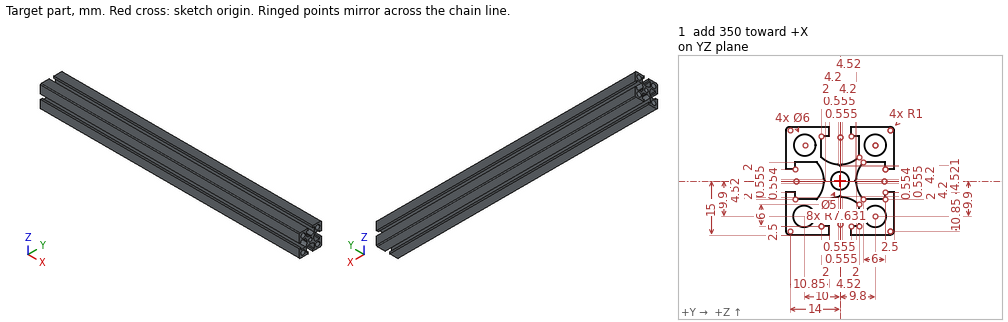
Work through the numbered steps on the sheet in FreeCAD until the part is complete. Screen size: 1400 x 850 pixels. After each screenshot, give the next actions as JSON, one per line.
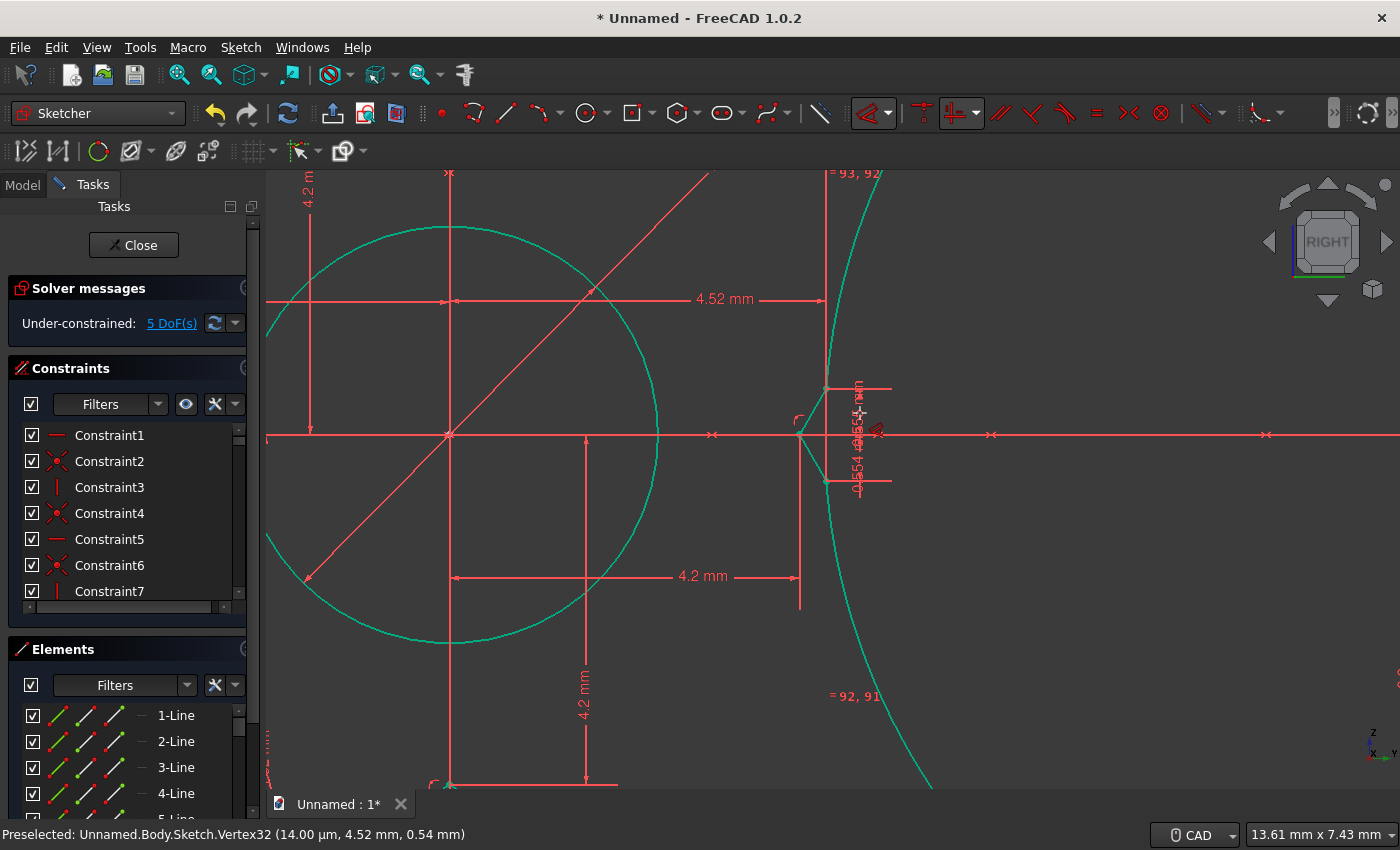
{"action": "scroll", "coordinate": [827, 488], "scroll_direction": "down", "scroll_amount": 9}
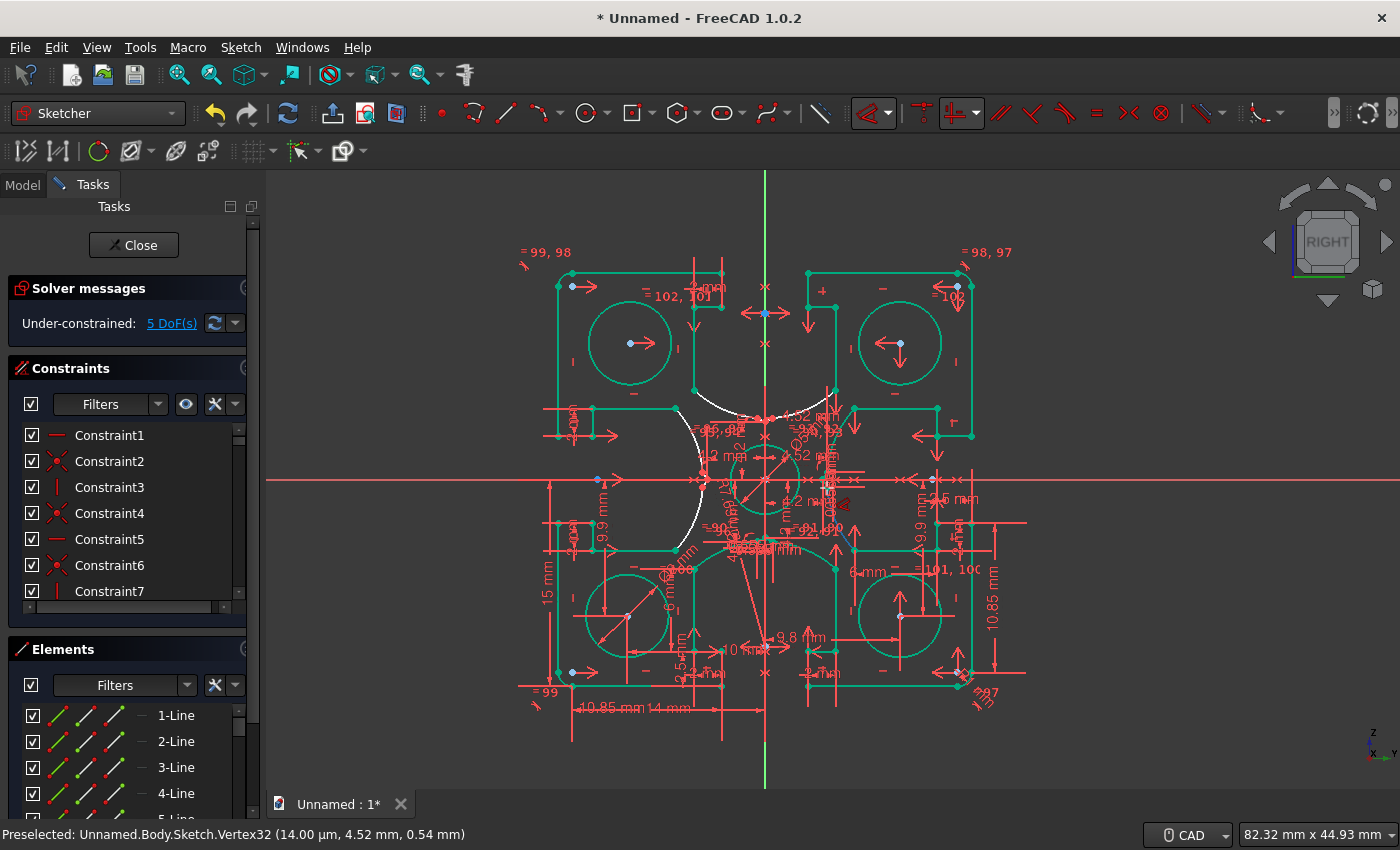
{"action": "scroll", "coordinate": [772, 418], "scroll_direction": "up", "scroll_amount": 9}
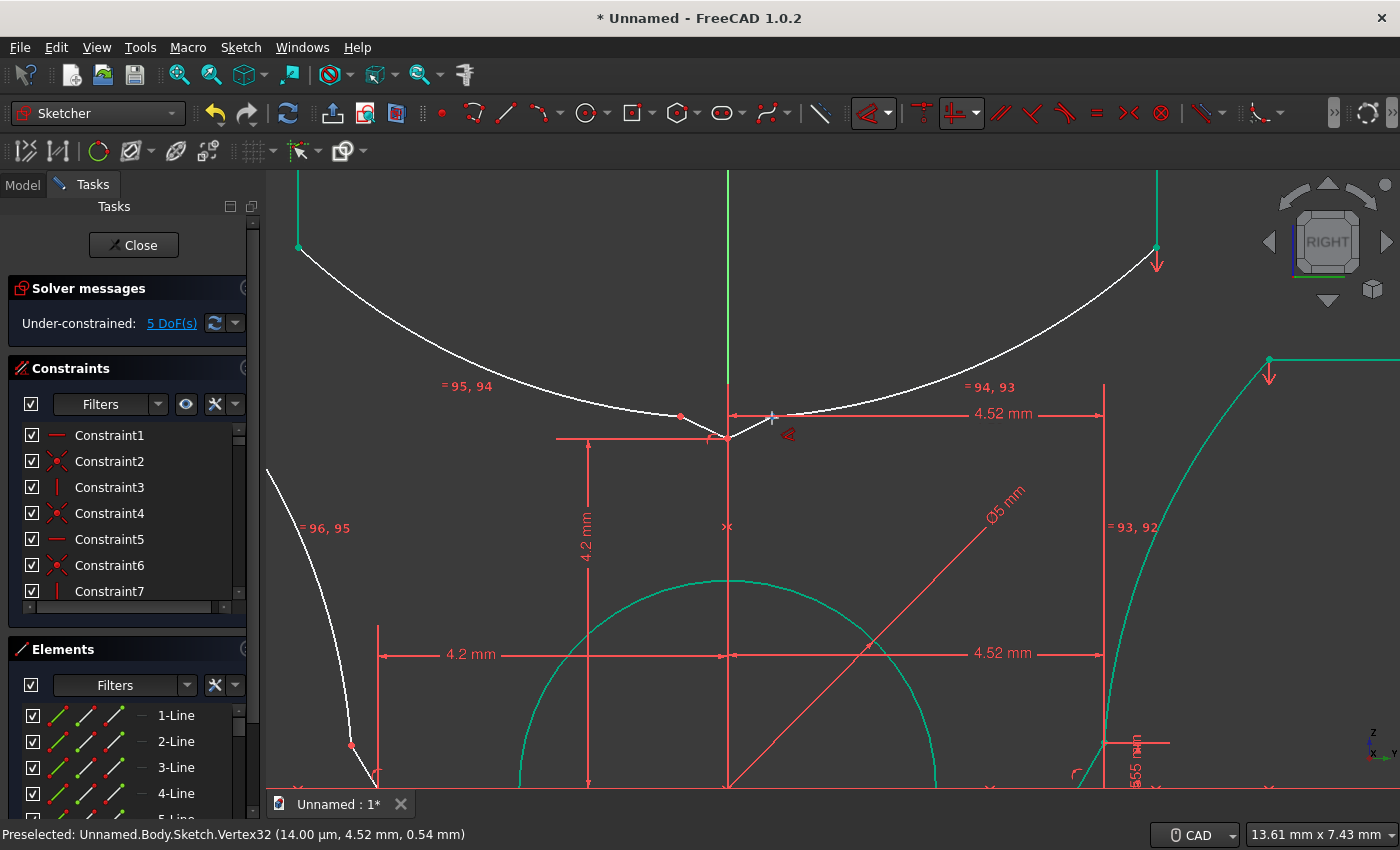
{"action": "left_click", "coordinate": [772, 417]}
{"action": "left_click", "coordinate": [750, 383]}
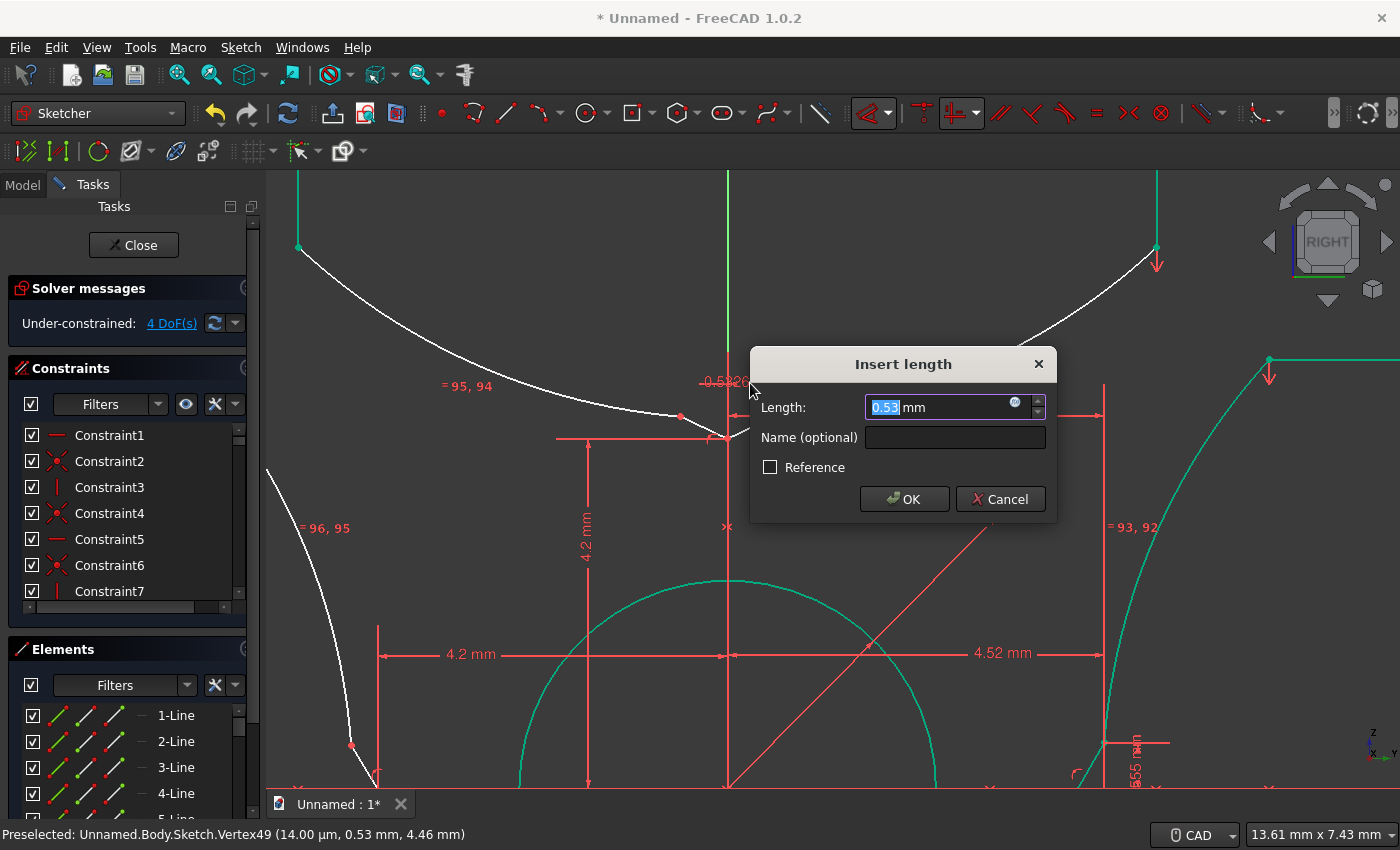
{"action": "type", "text": "0.555"}
{"action": "key", "text": "Return"}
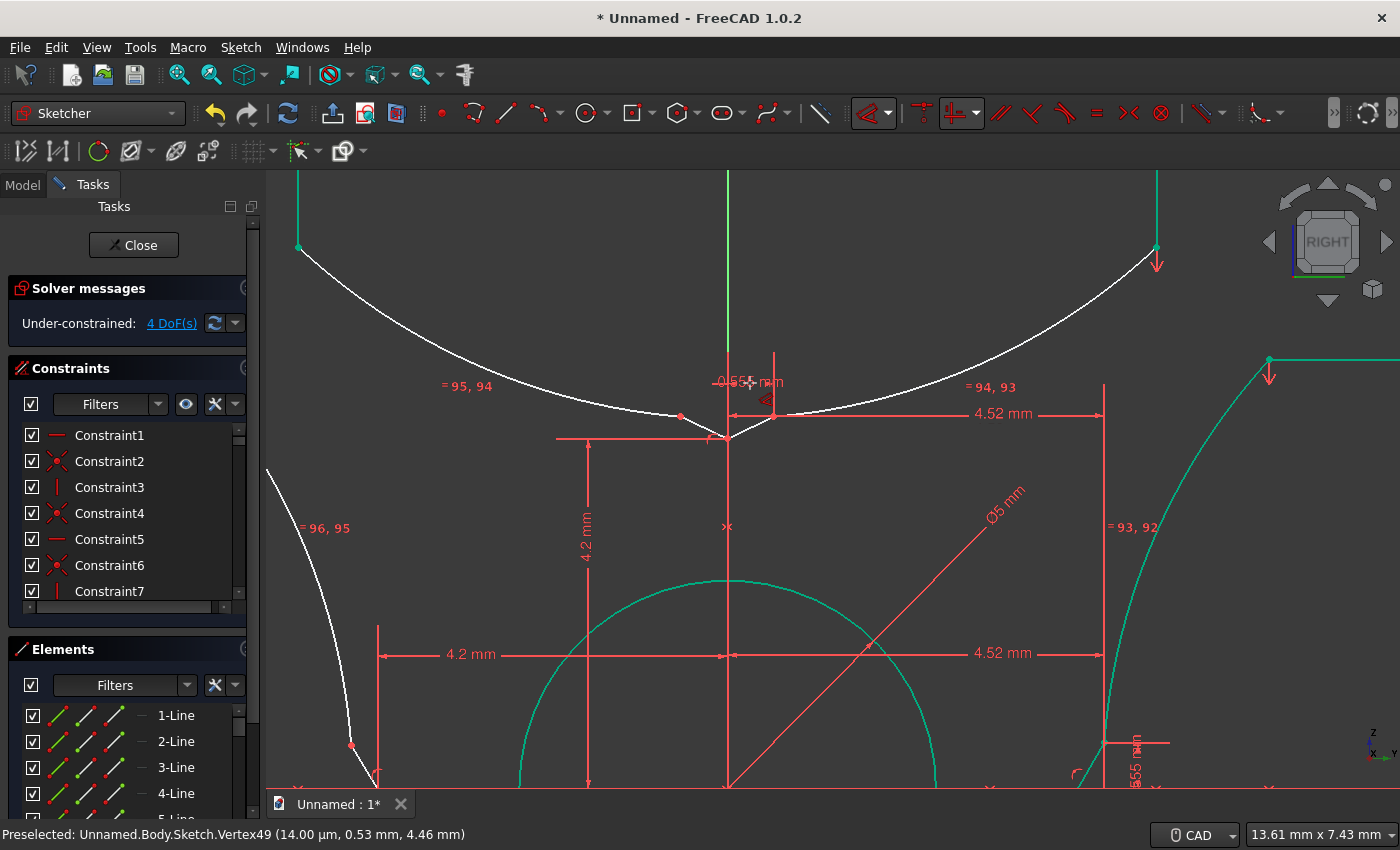
{"action": "scroll", "coordinate": [772, 418], "scroll_direction": "down", "scroll_amount": 9}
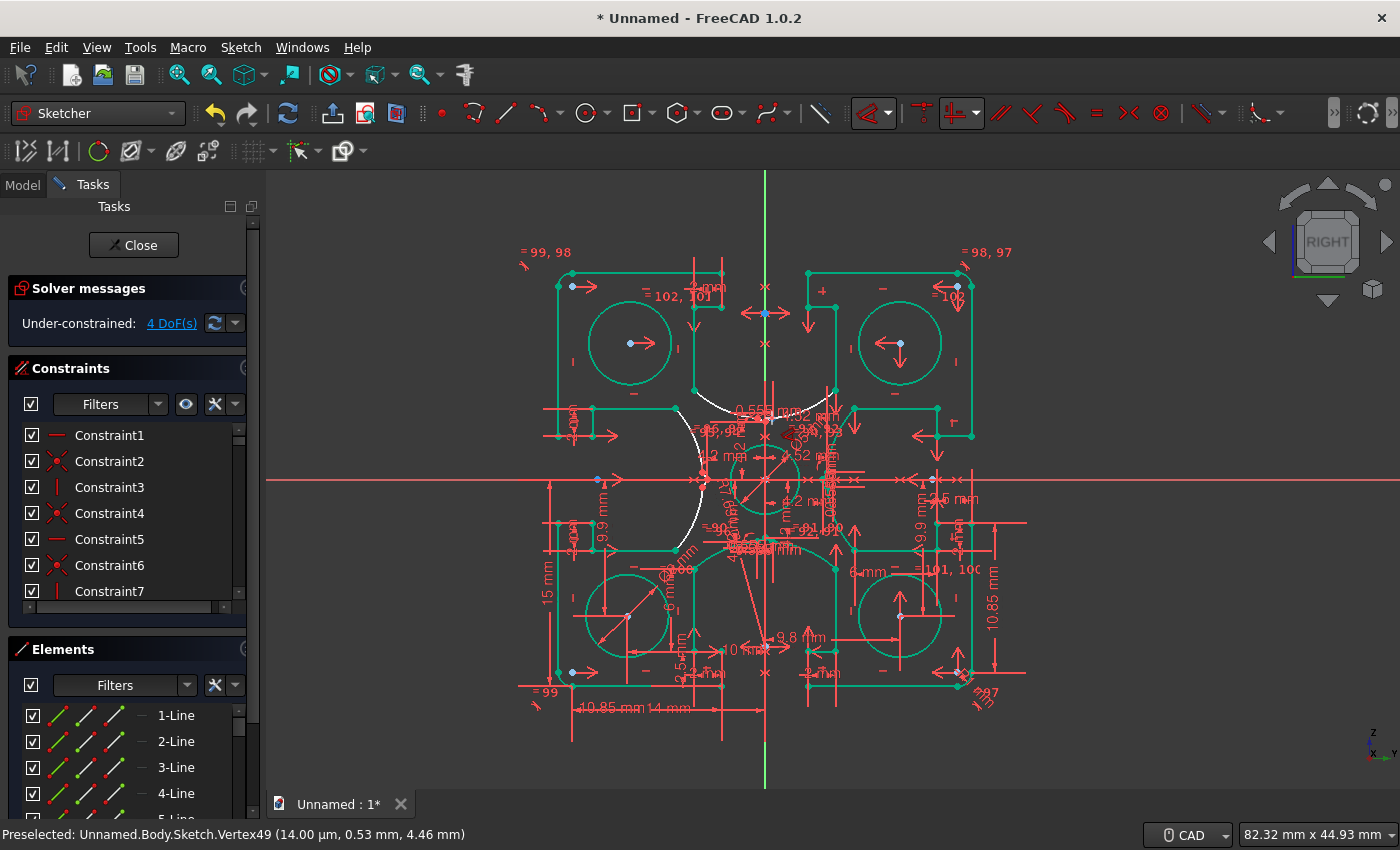
{"action": "scroll", "coordinate": [773, 418], "scroll_direction": "up", "scroll_amount": 2}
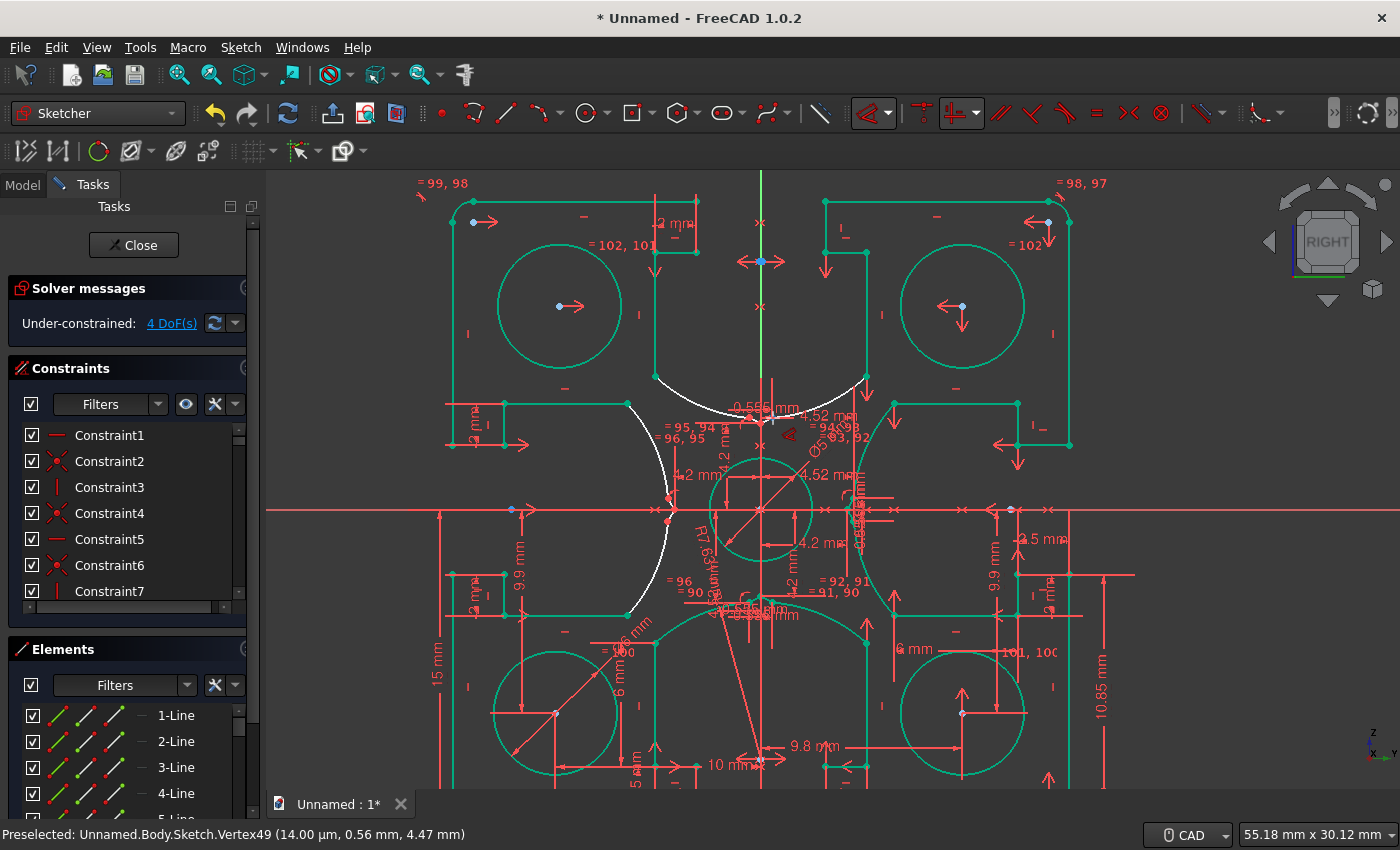
{"action": "left_click", "coordinate": [772, 418]}
{"action": "left_click", "coordinate": [727, 496]}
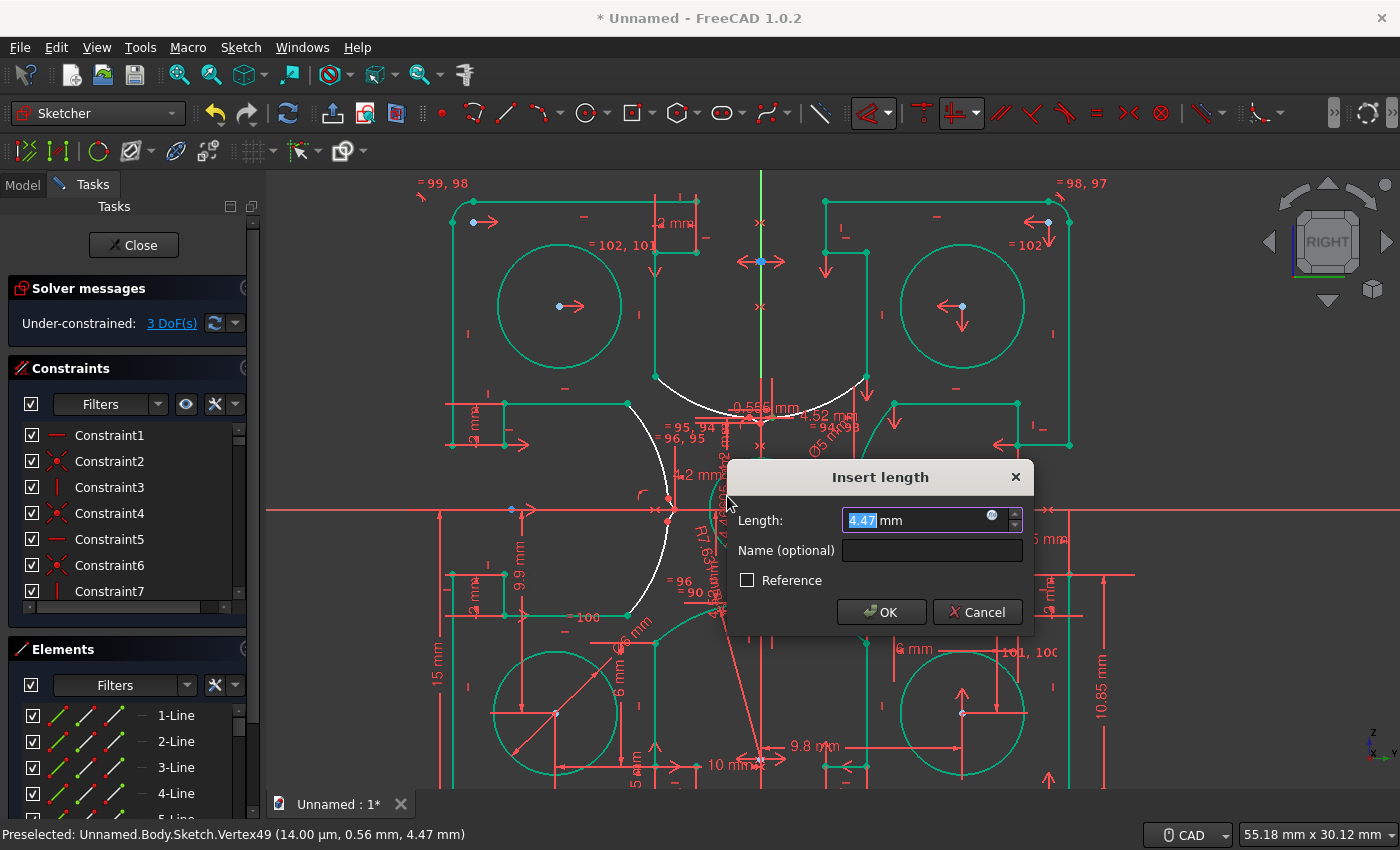
{"action": "type", "text": "4.521"}
{"action": "key", "text": "Return"}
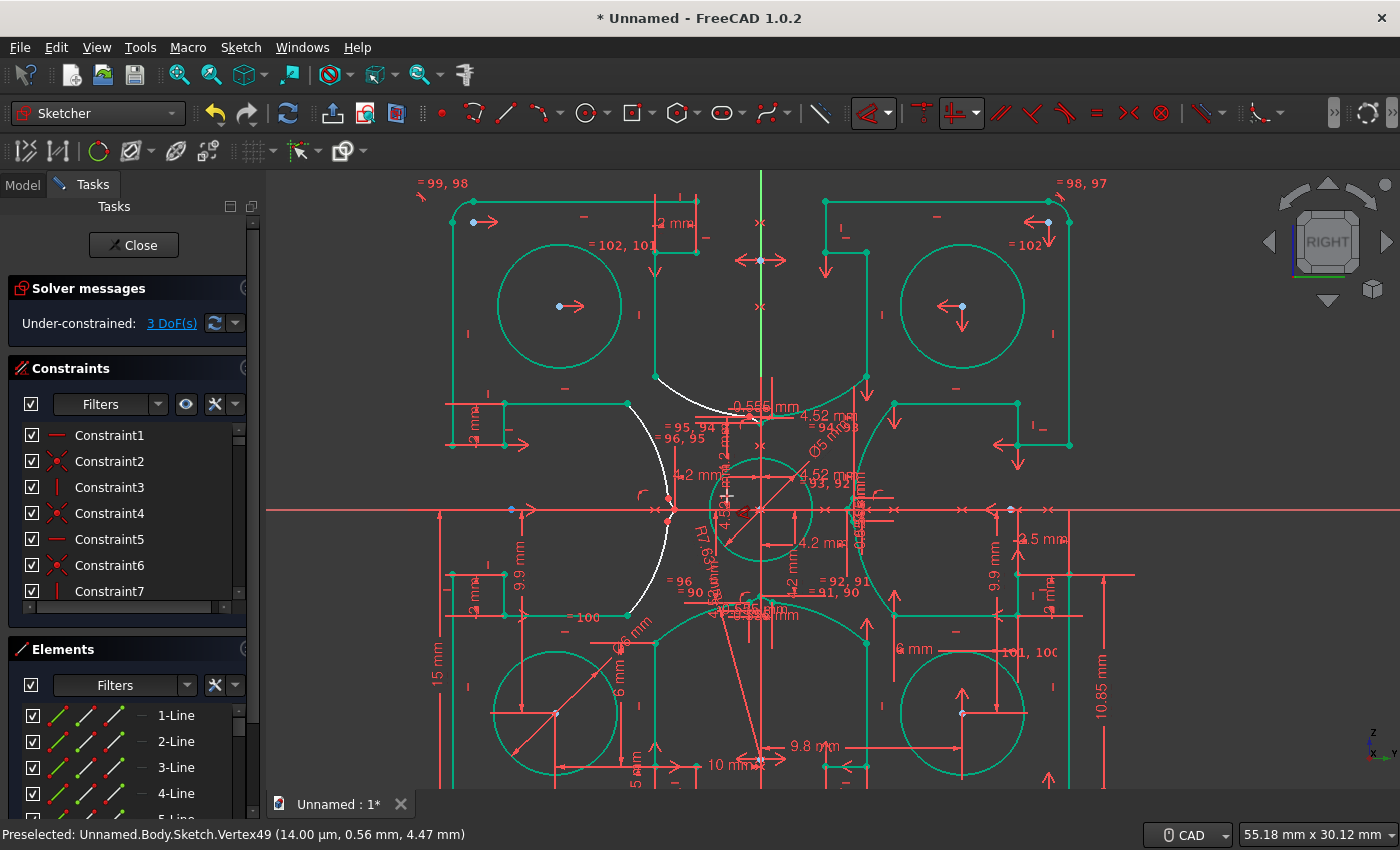
{"action": "scroll", "coordinate": [749, 417], "scroll_direction": "up", "scroll_amount": 7}